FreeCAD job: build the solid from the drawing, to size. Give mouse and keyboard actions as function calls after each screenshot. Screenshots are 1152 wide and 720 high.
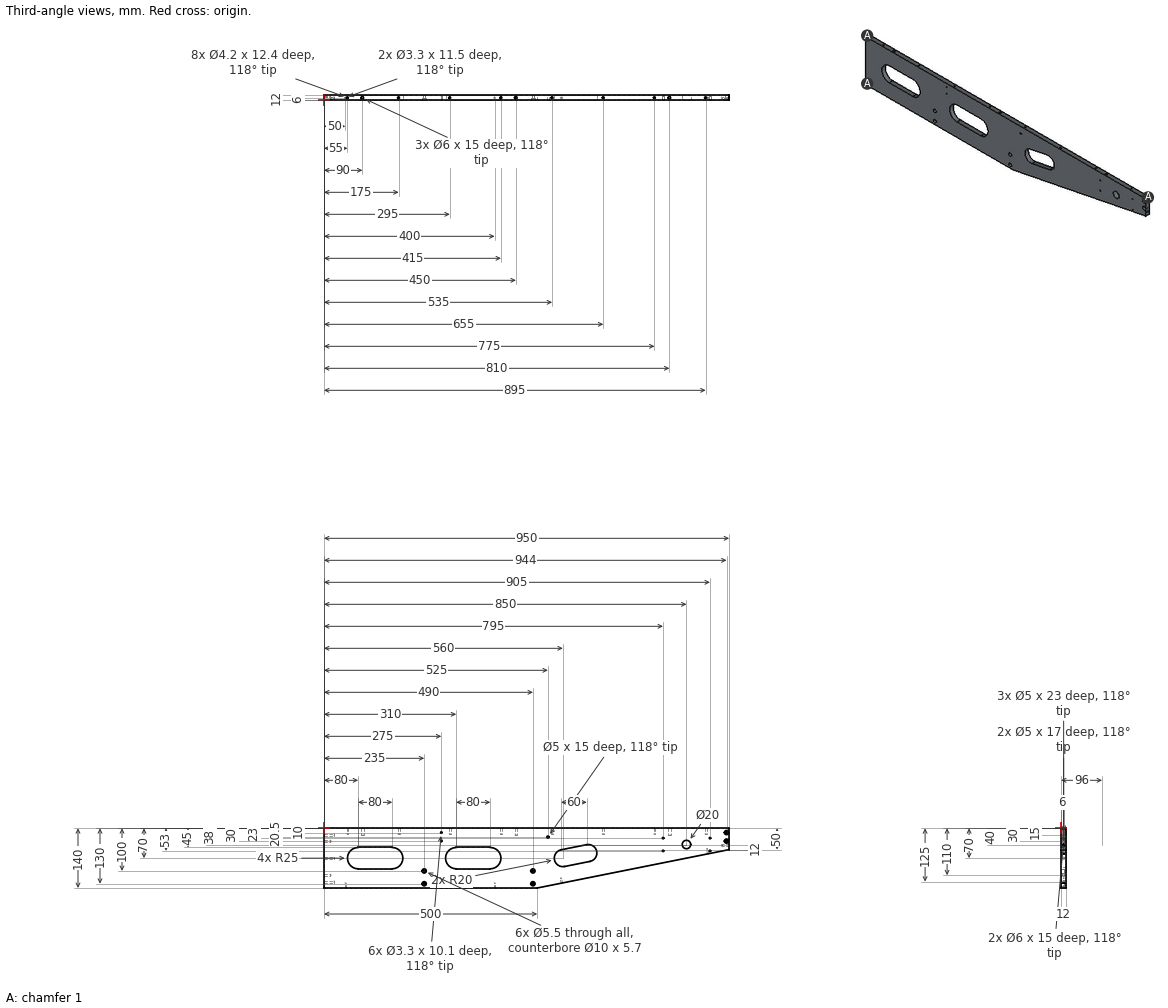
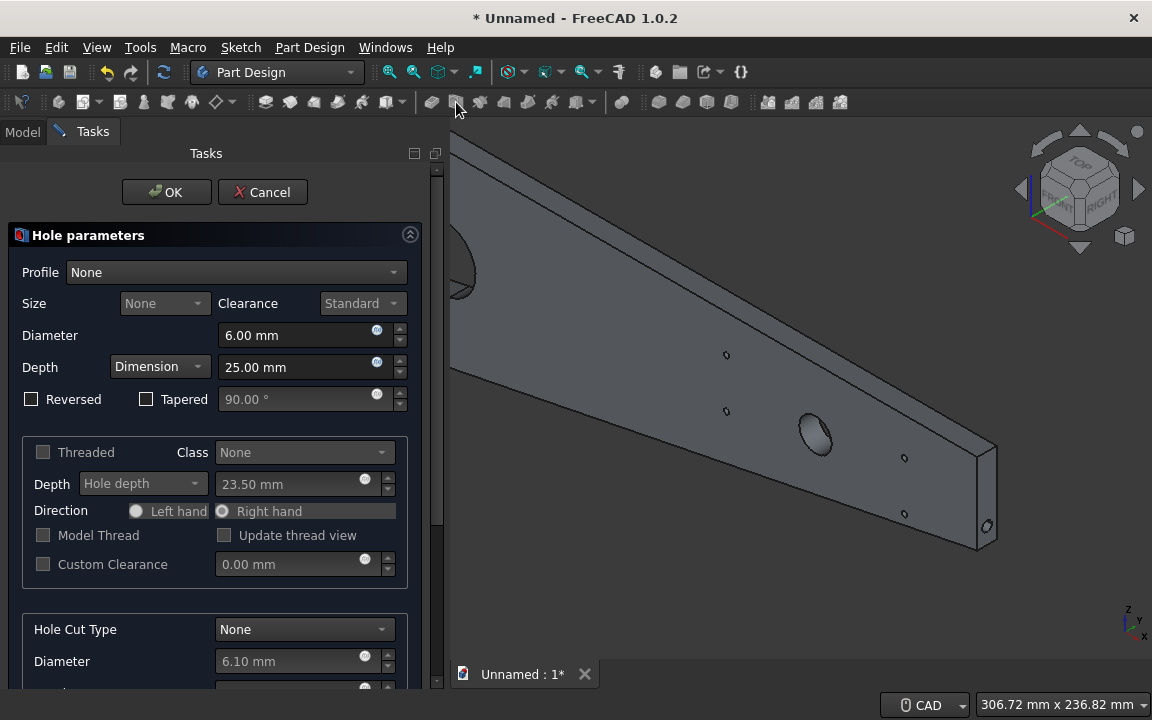
triple_click(305, 335)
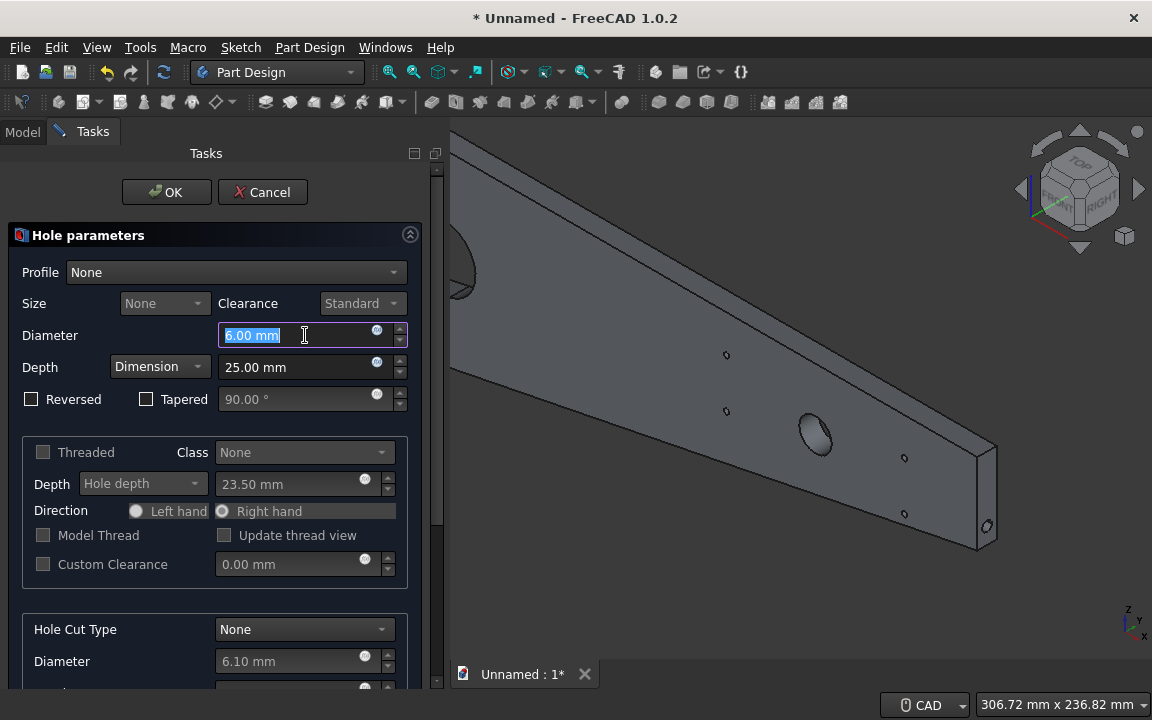
text(5)
key(Tab)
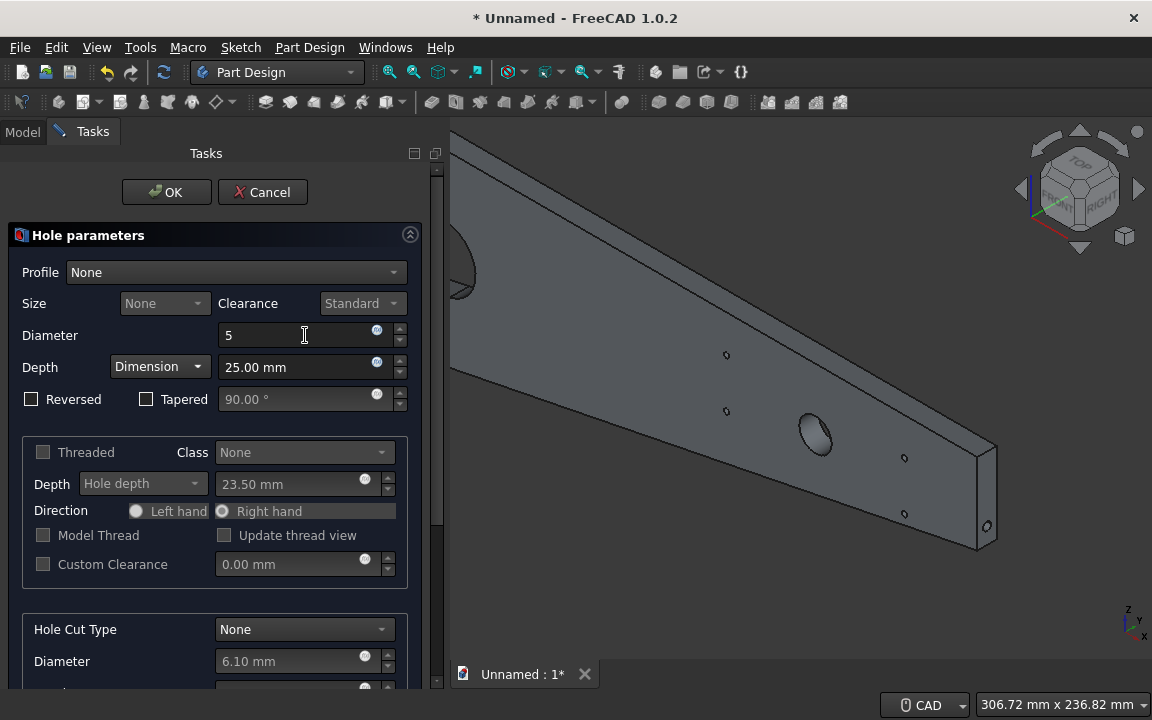
triple_click(305, 367)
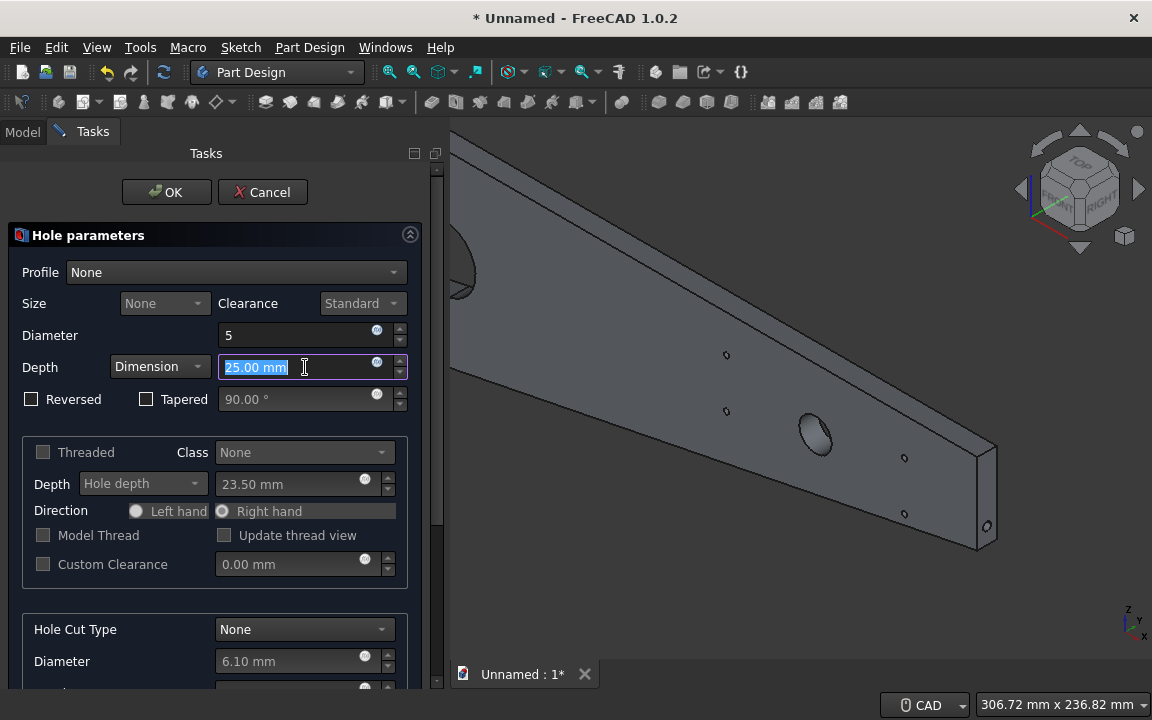
text(17)
key(Tab)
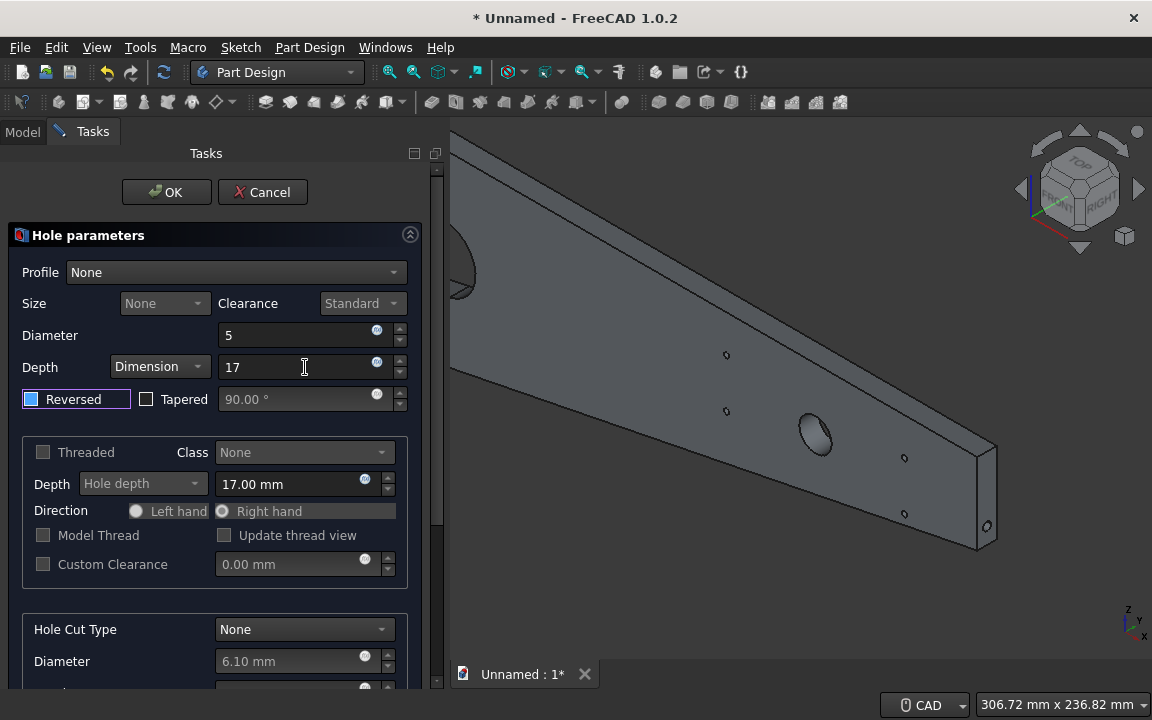
click(167, 192)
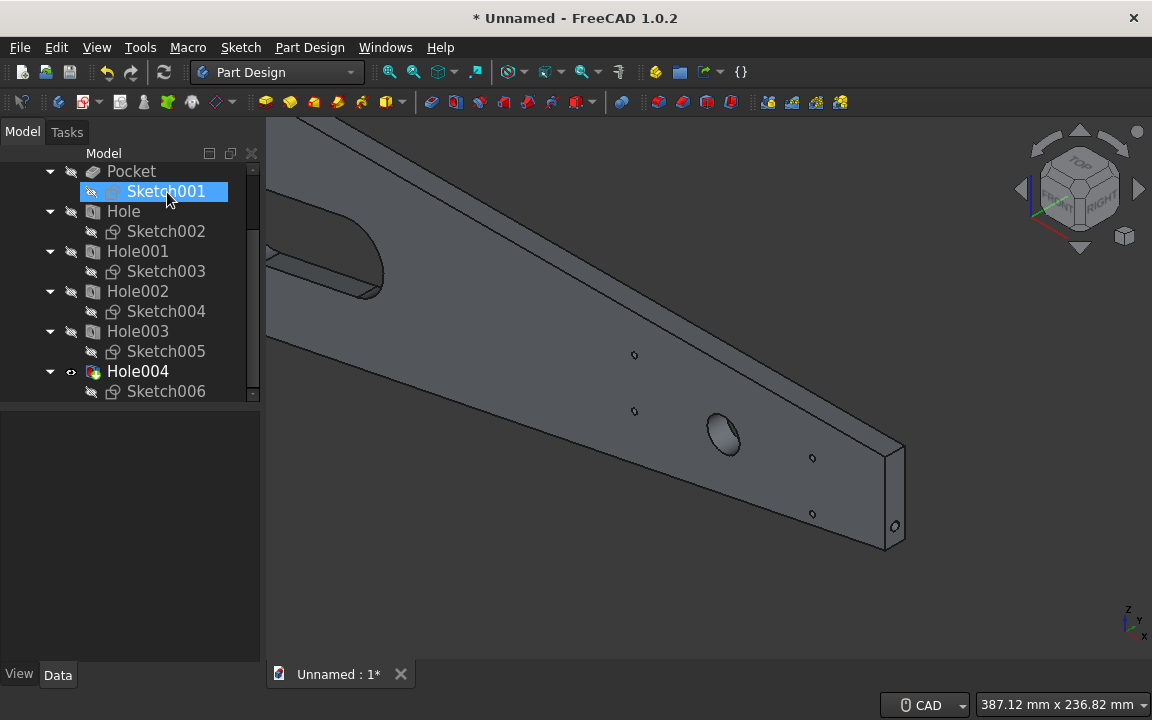
key(v)
key(f)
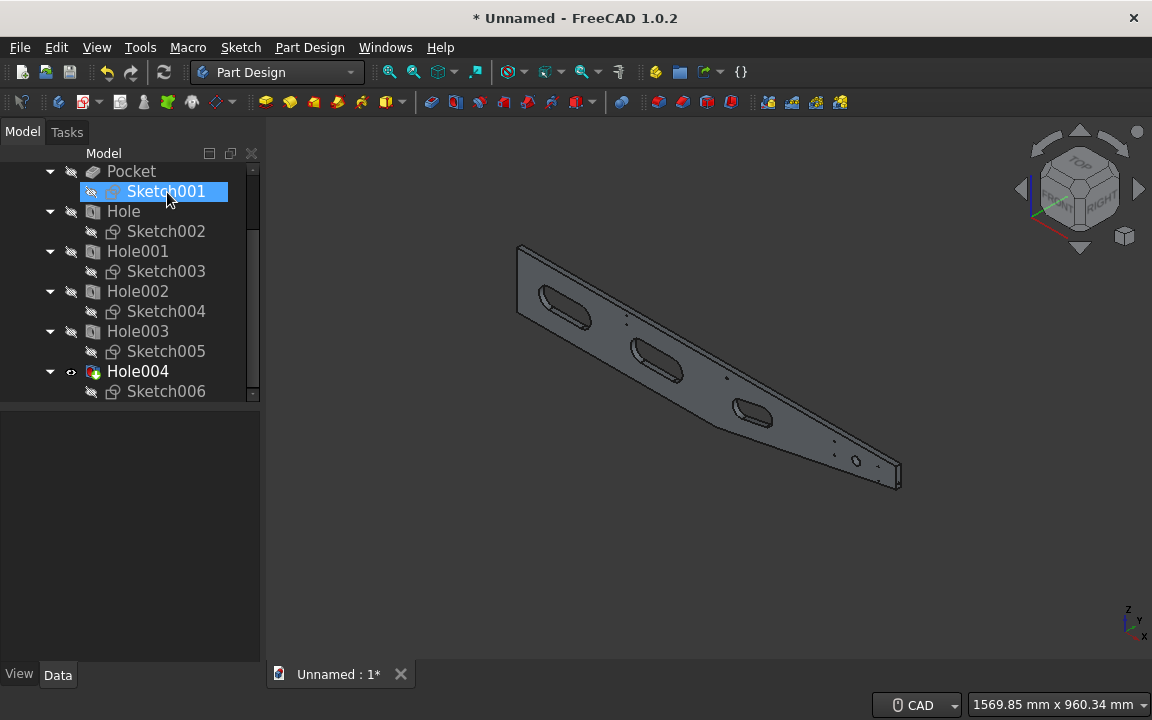
key(6)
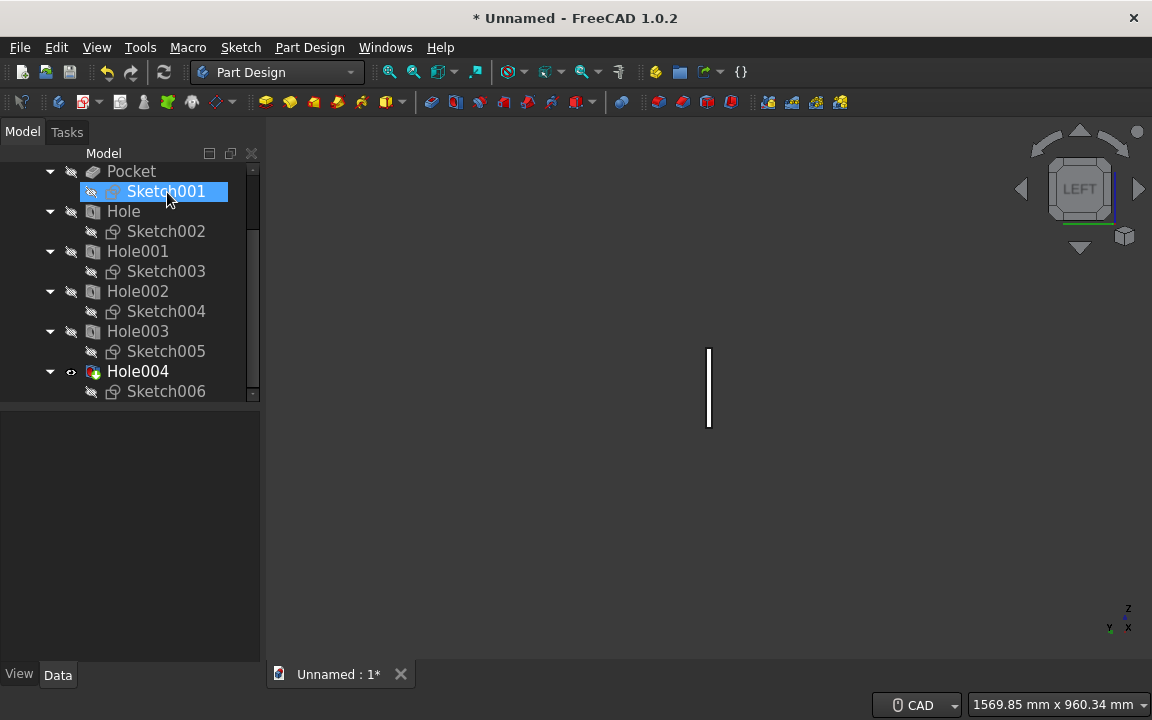
key(v)
key(f)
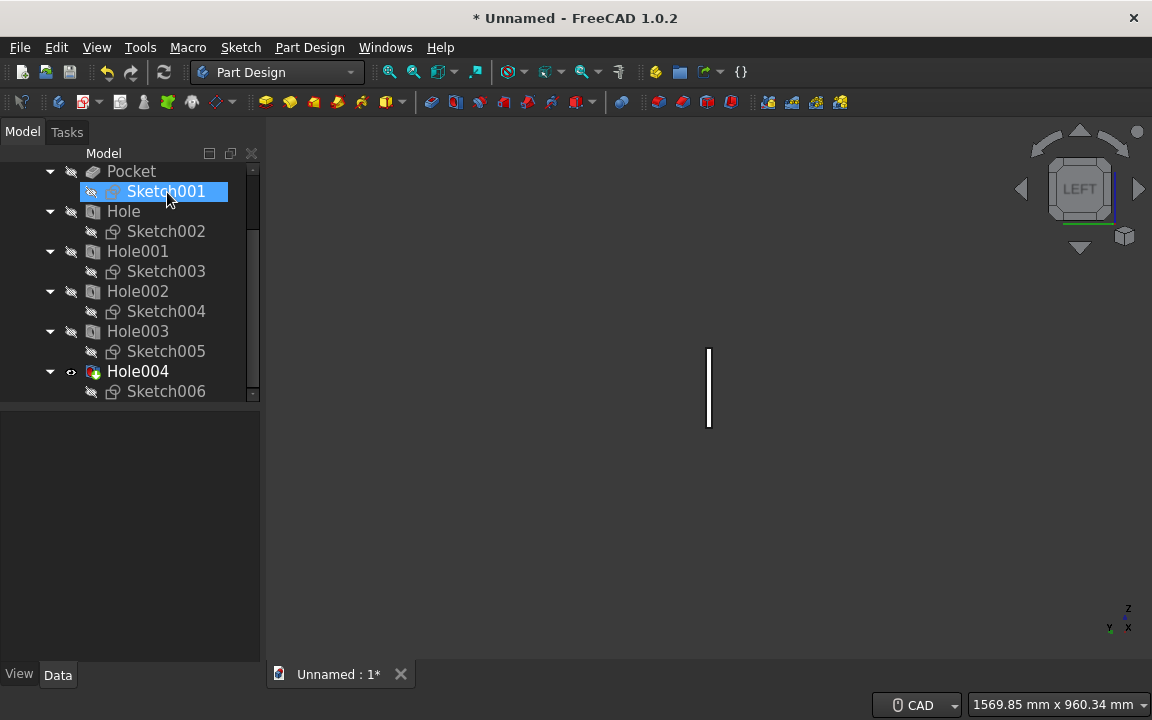
scroll(709, 353, up, 7)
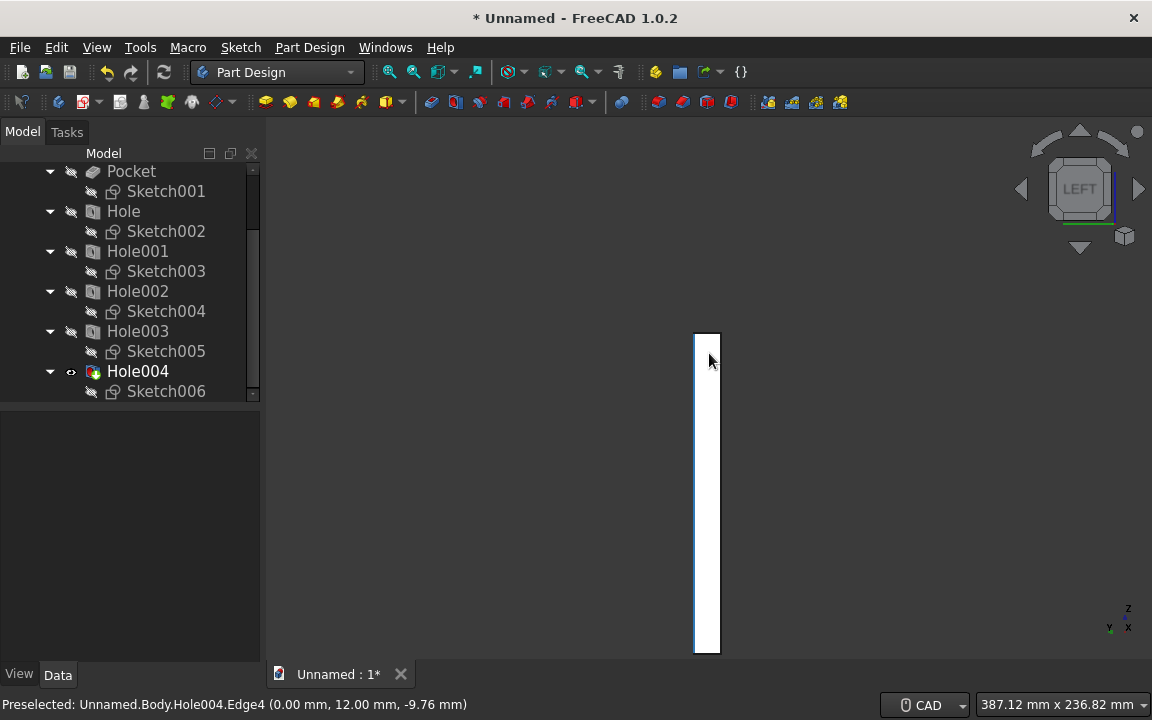
click(707, 355)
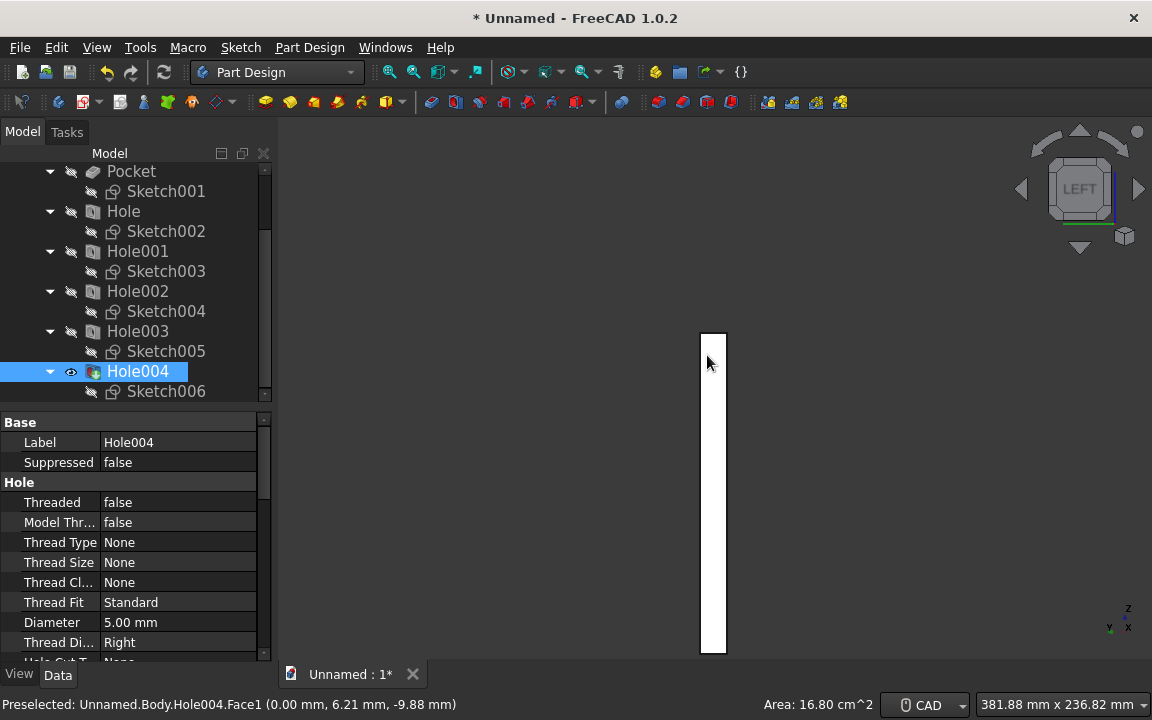
click(84, 102)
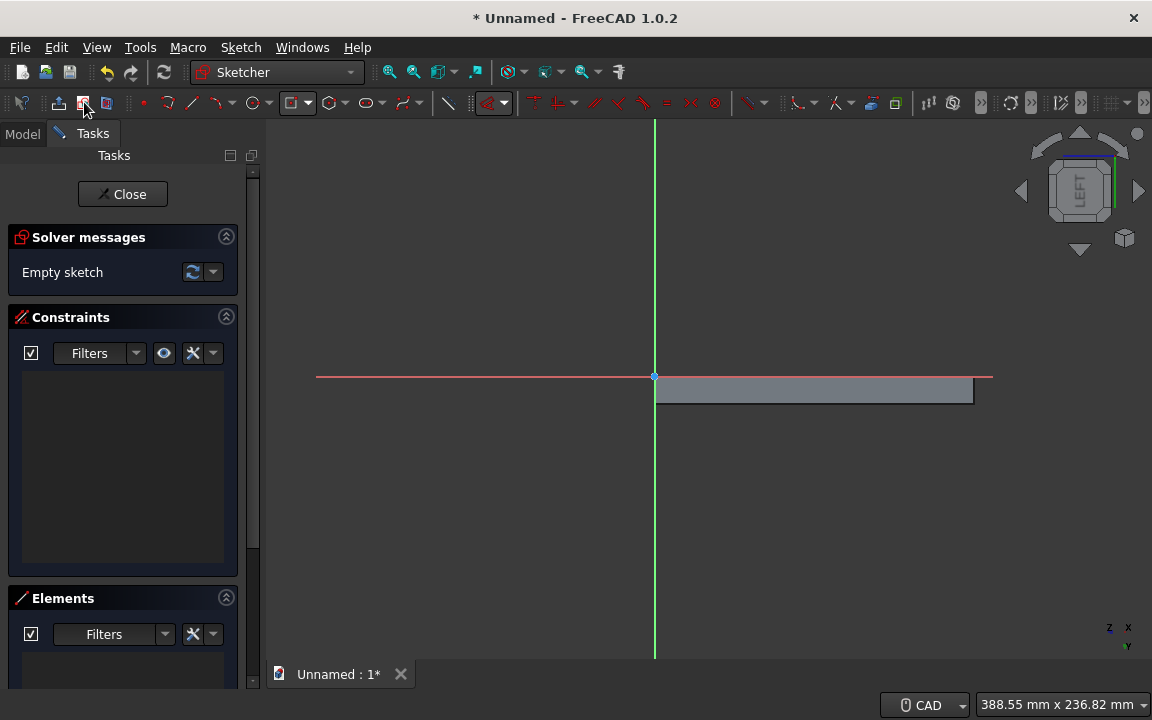
scroll(987, 384, up, 3)